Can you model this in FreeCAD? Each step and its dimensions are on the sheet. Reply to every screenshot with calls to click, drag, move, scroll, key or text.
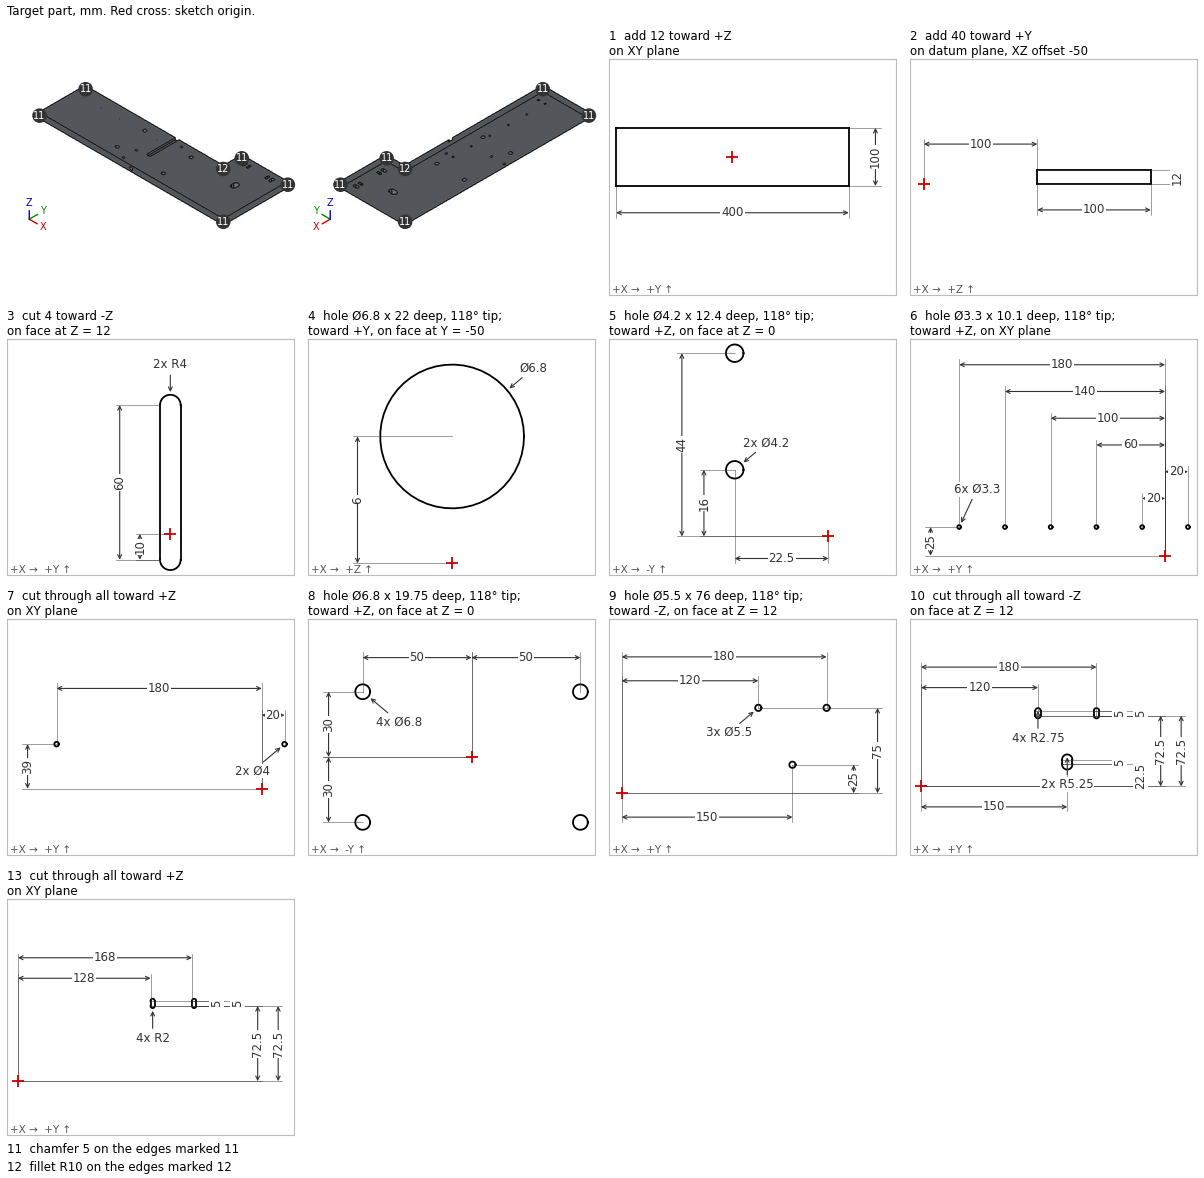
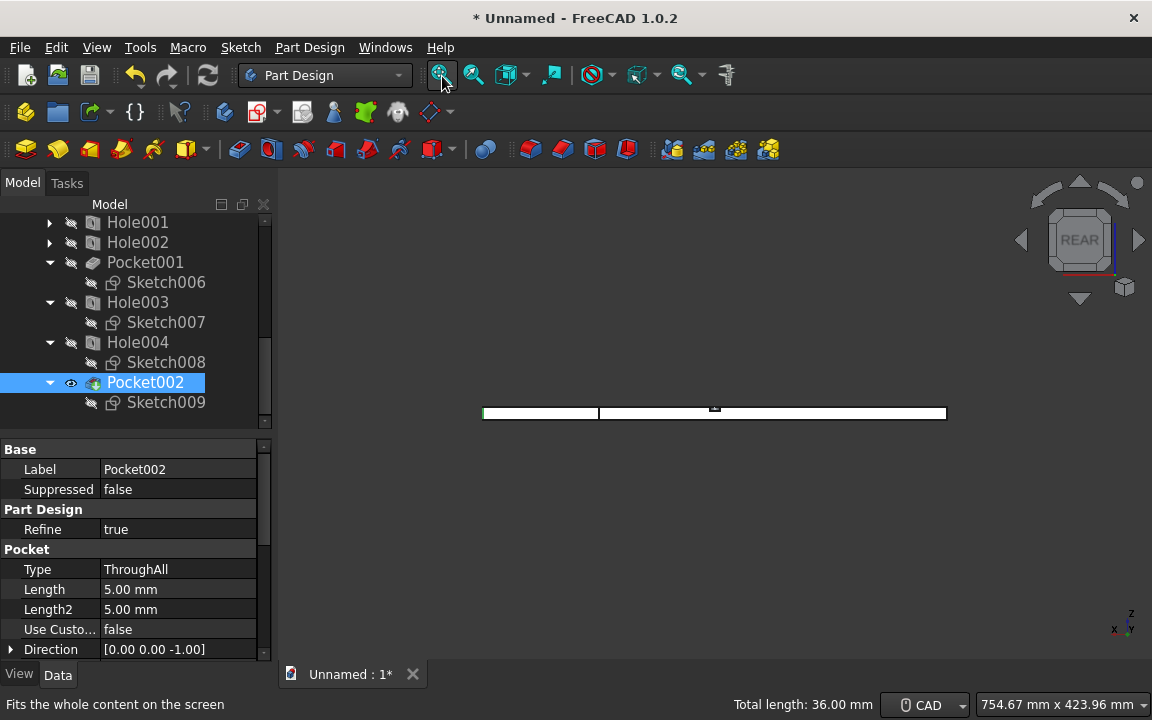
click(599, 412, ctrl)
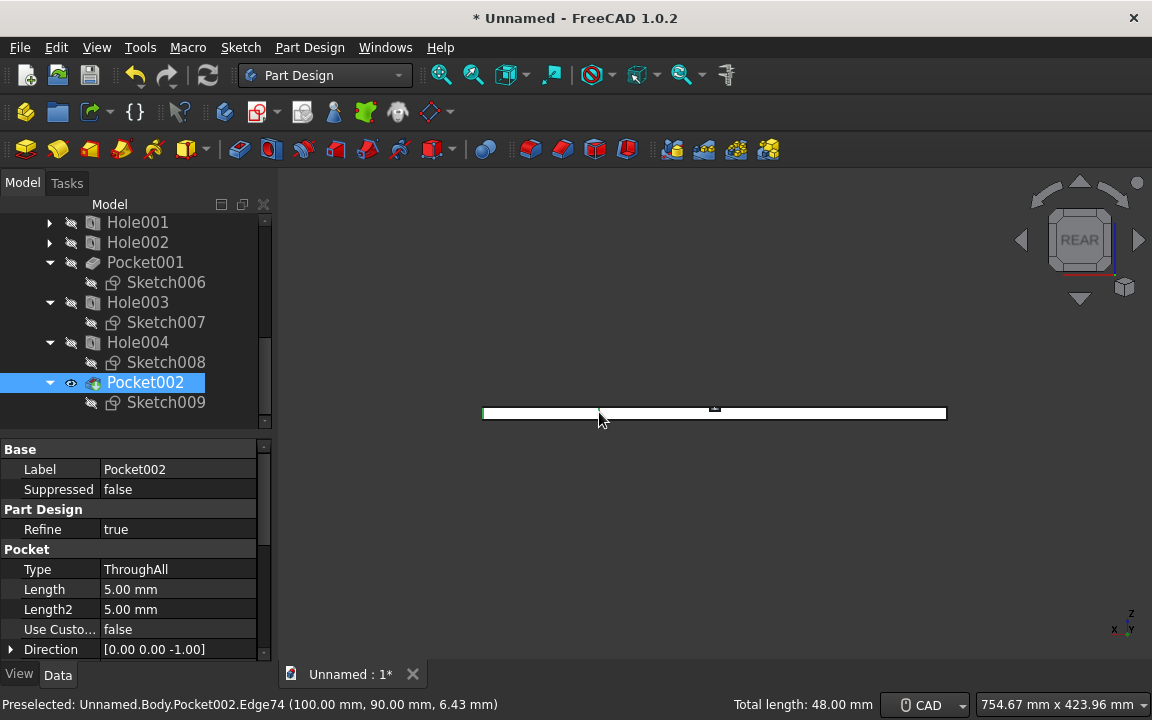
click(947, 412, ctrl)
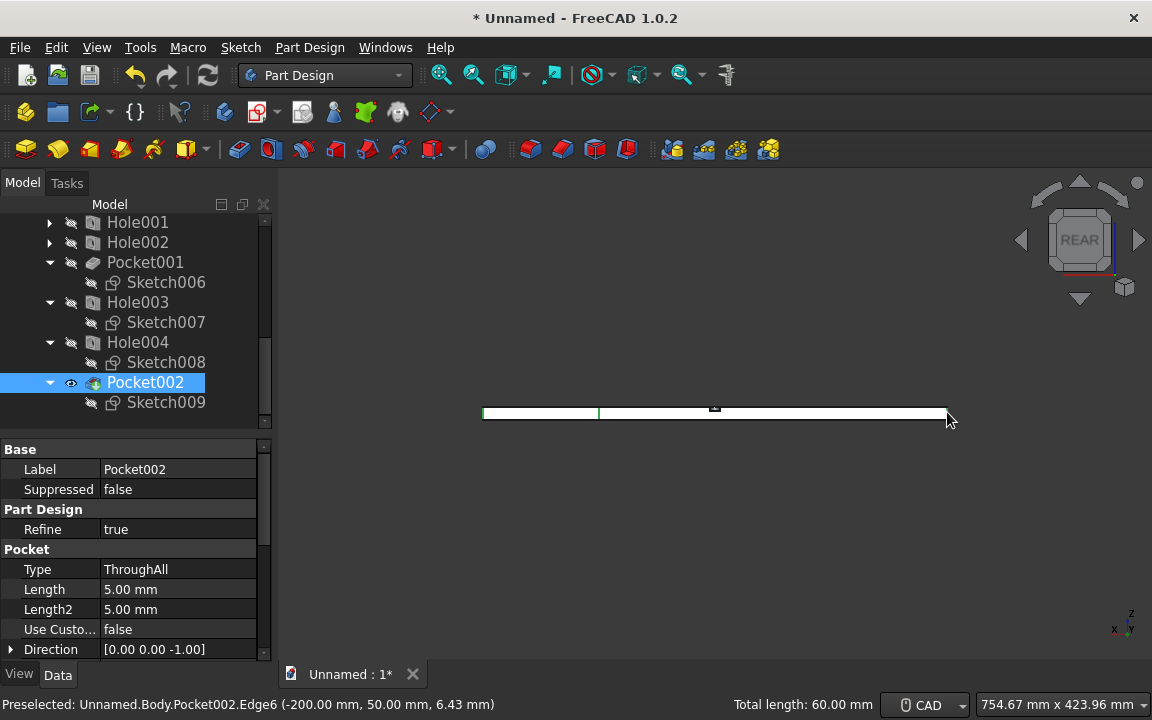
click(564, 150)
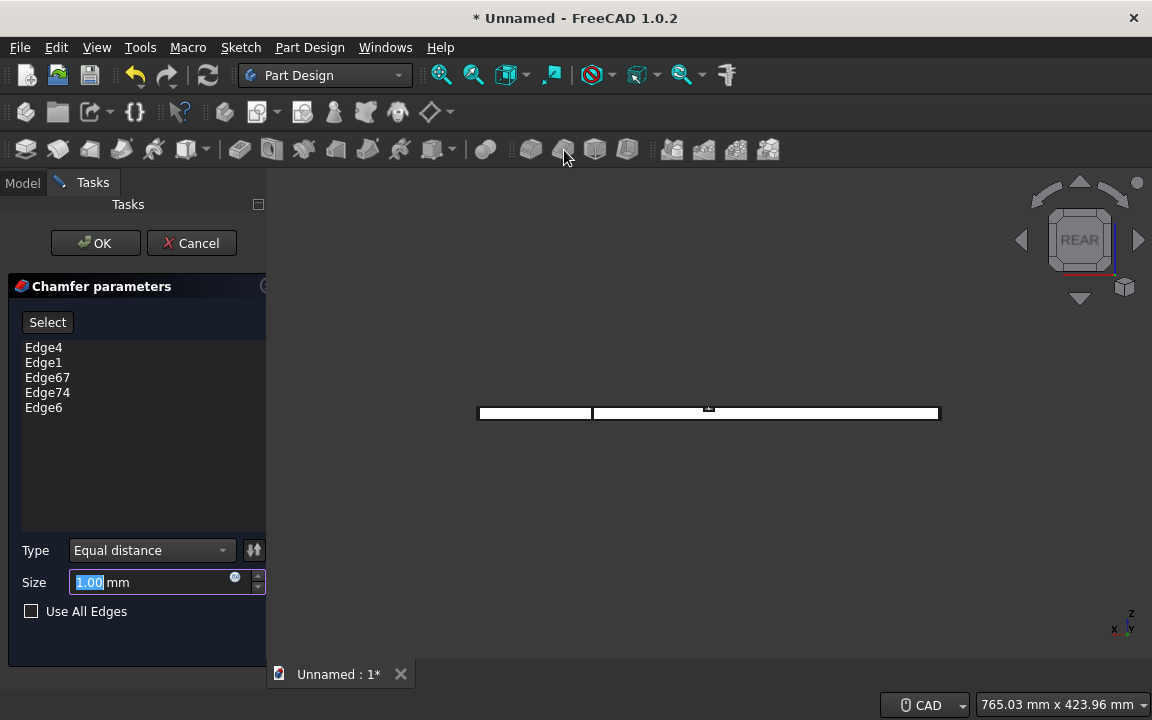
text(5)
key(Tab)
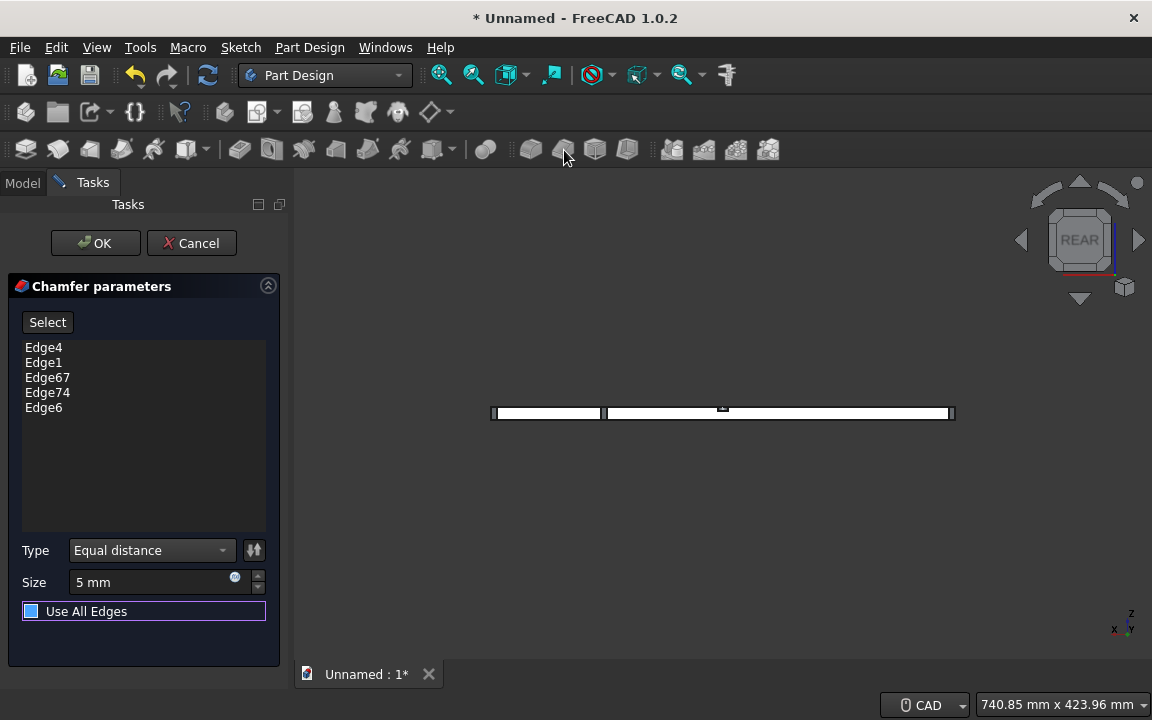
click(96, 243)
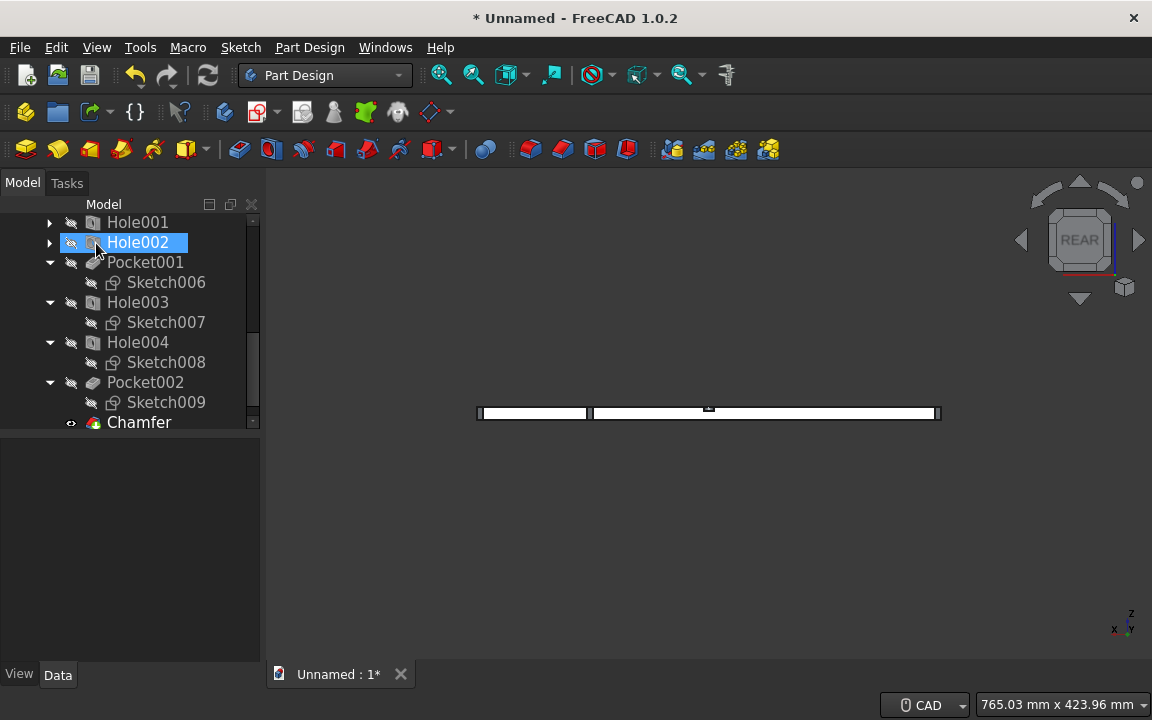
scroll(593, 412, up, 6)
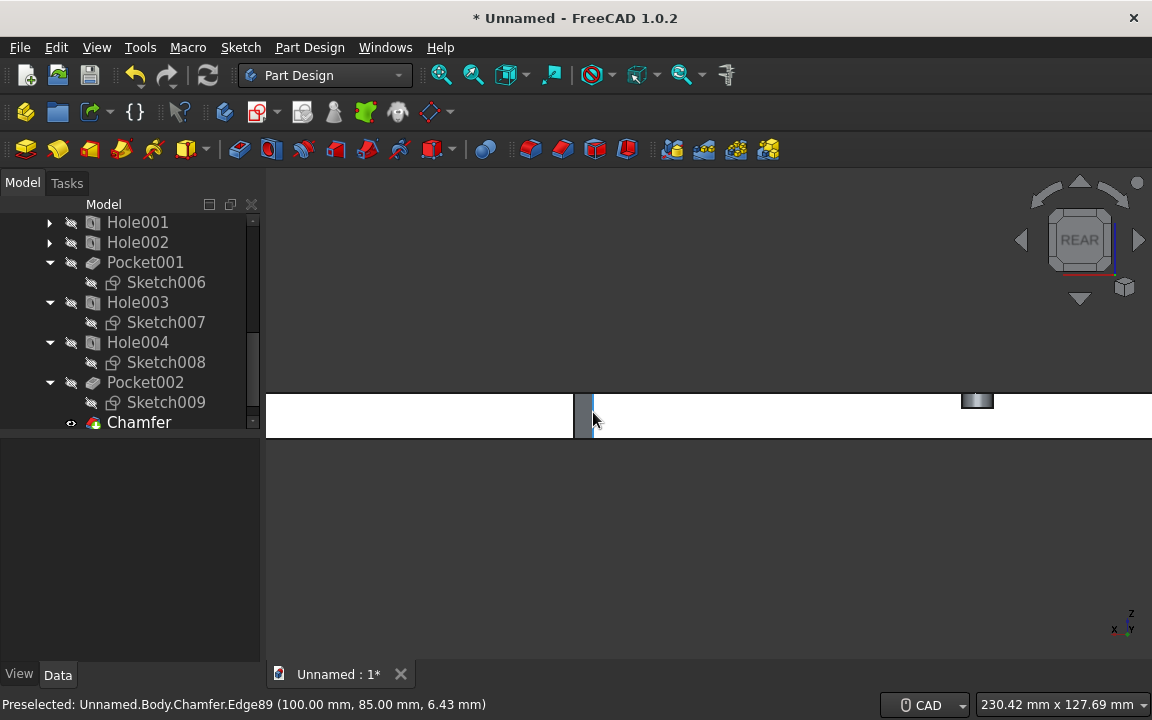
click(442, 76)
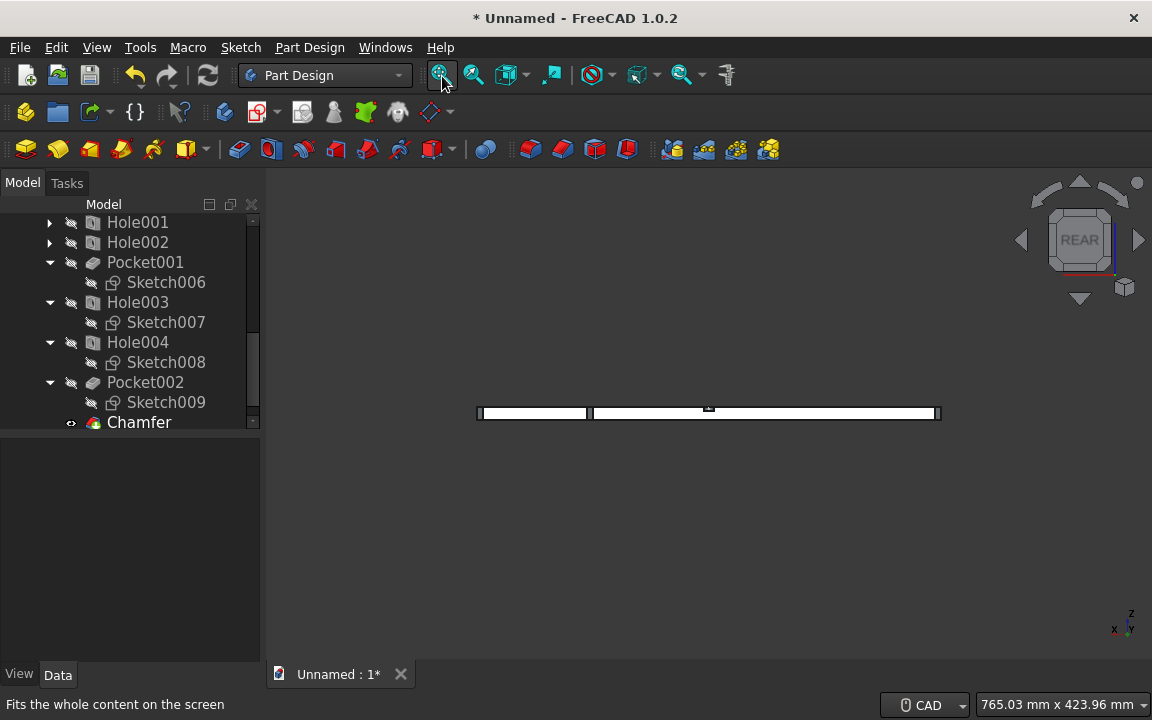
key(0)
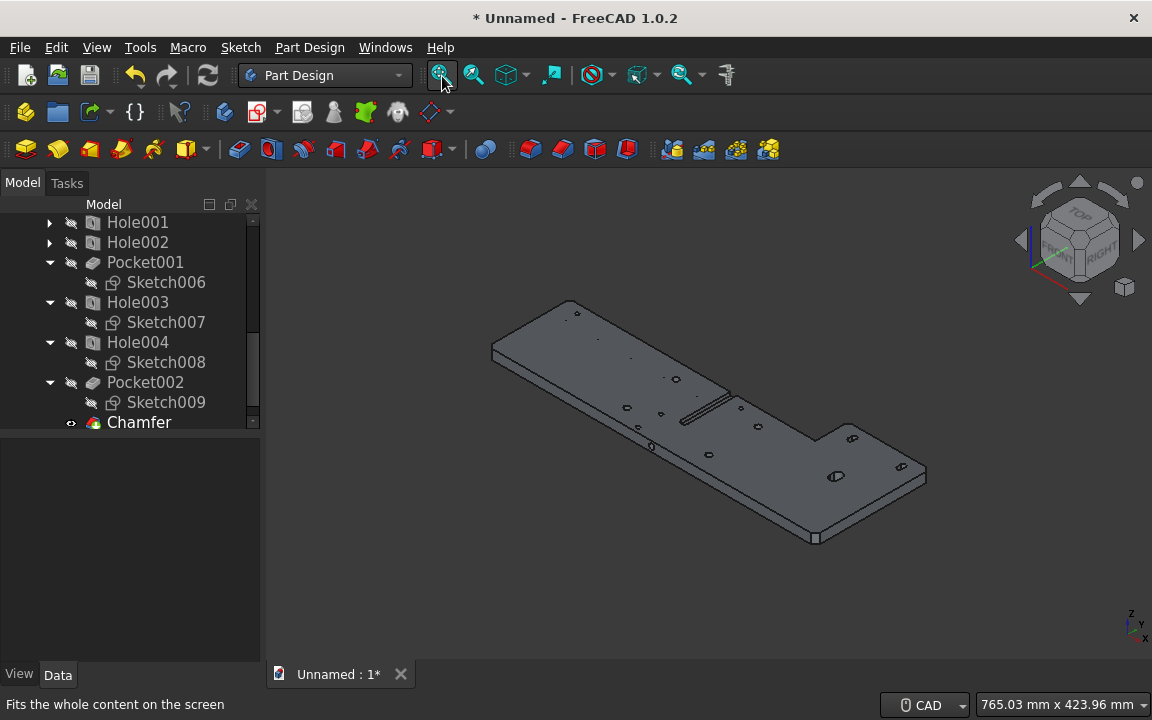
scroll(815, 446, up, 6)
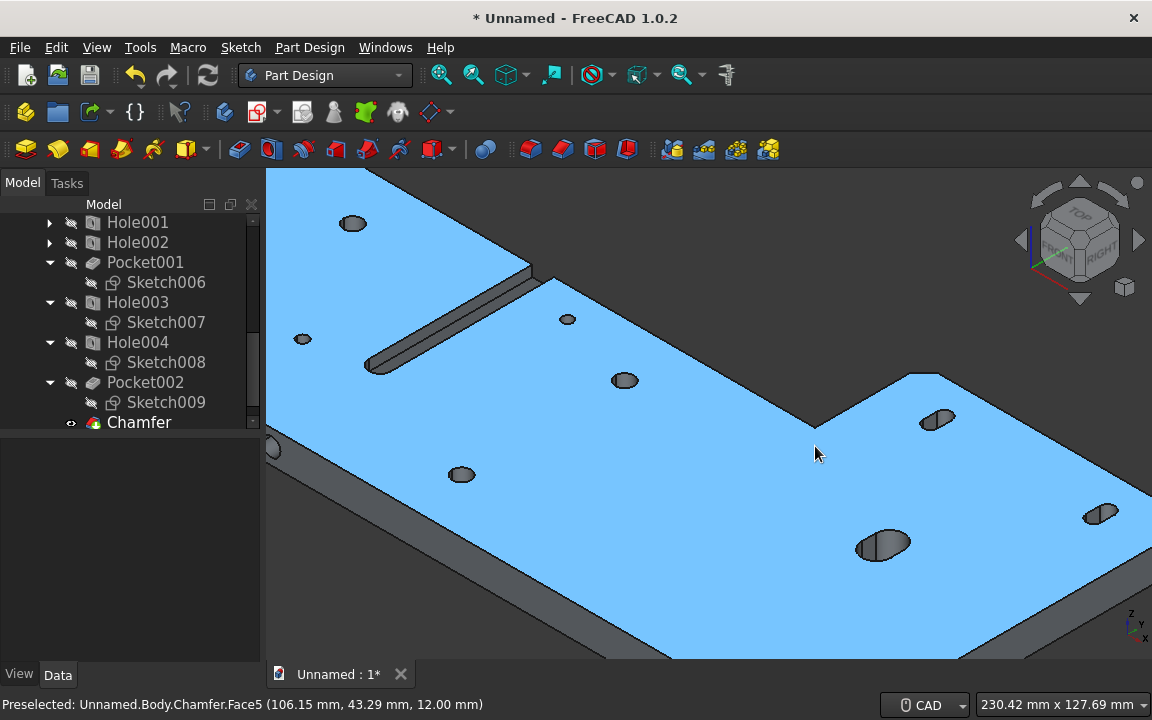
click(442, 76)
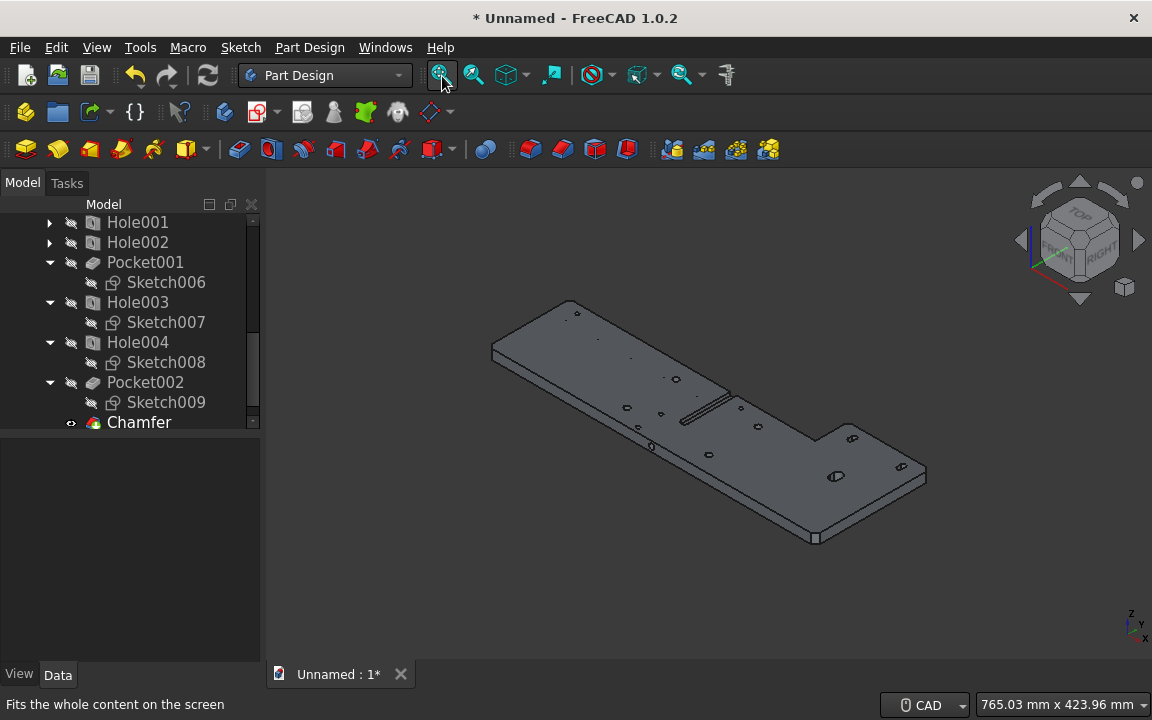
key(2)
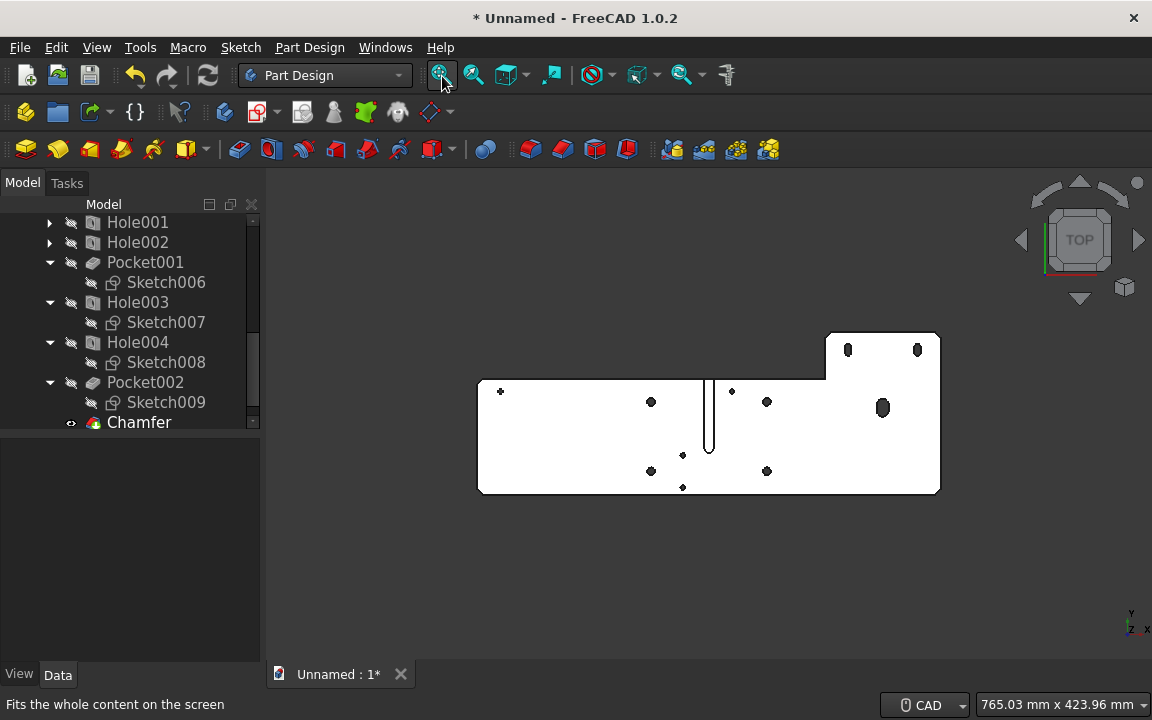
scroll(825, 378, up, 6)